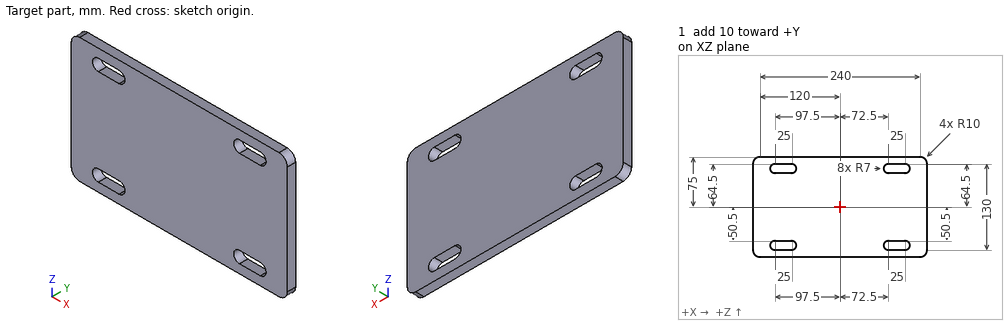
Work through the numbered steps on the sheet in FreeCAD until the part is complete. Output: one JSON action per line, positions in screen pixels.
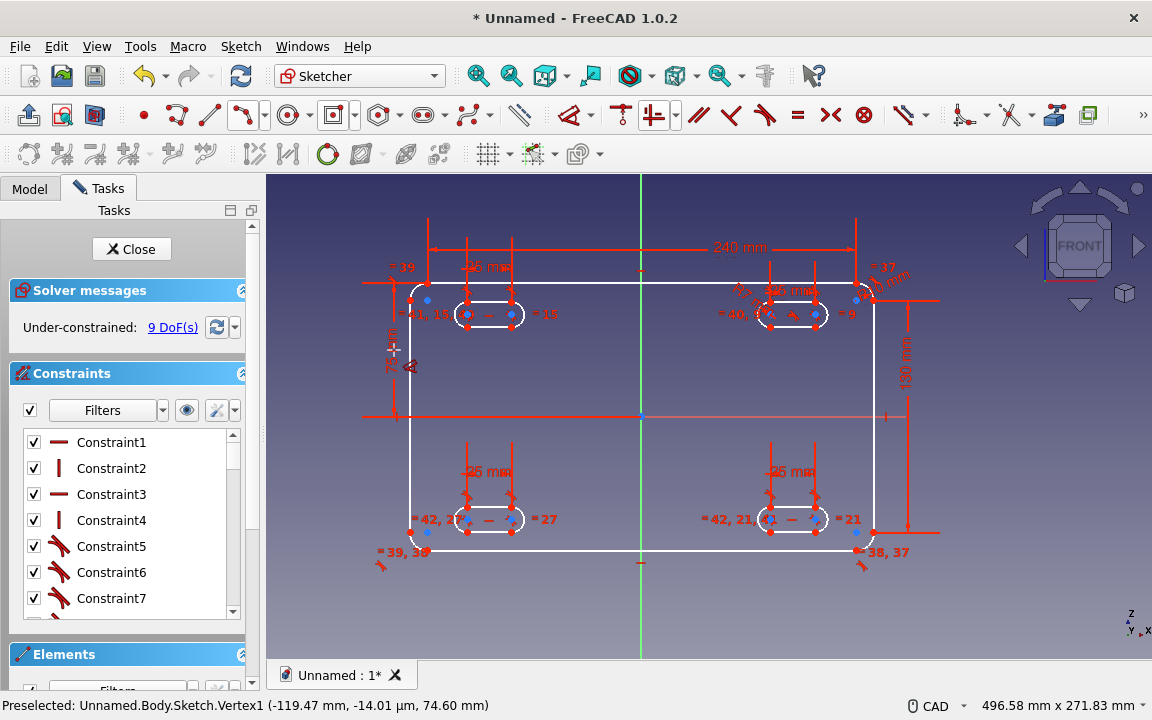
{"action": "left_click", "coordinate": [428, 283]}
{"action": "left_click", "coordinate": [583, 249]}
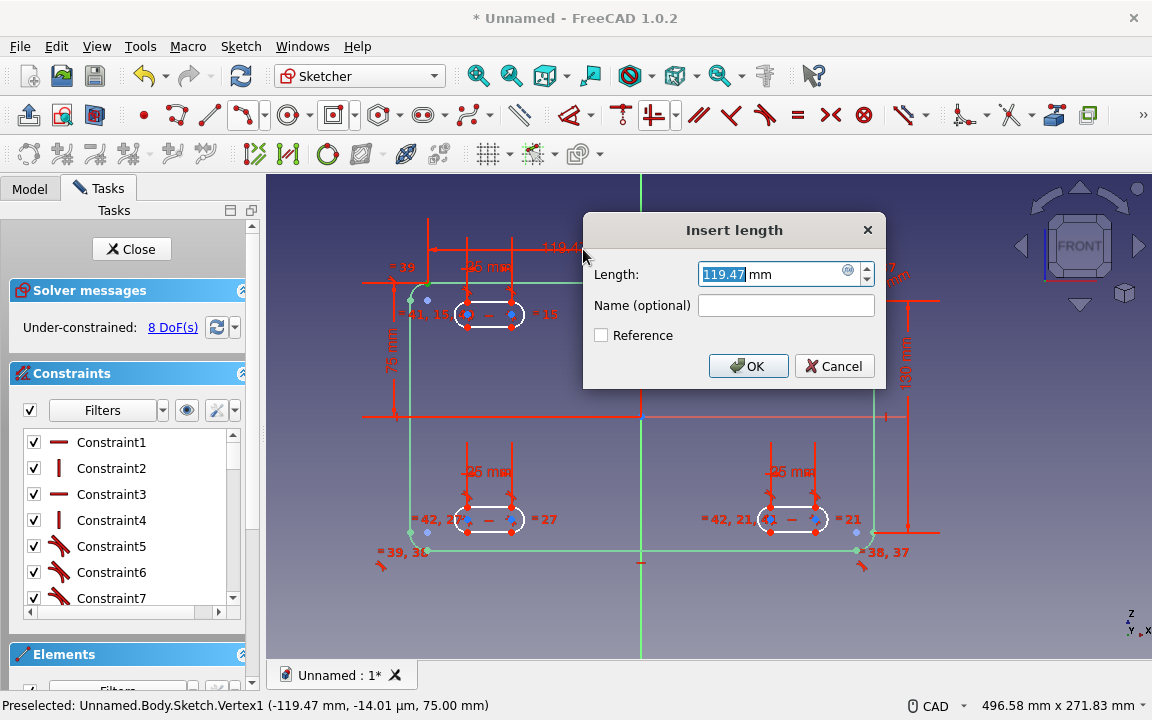
{"action": "type", "text": "120"}
{"action": "key", "text": "Return"}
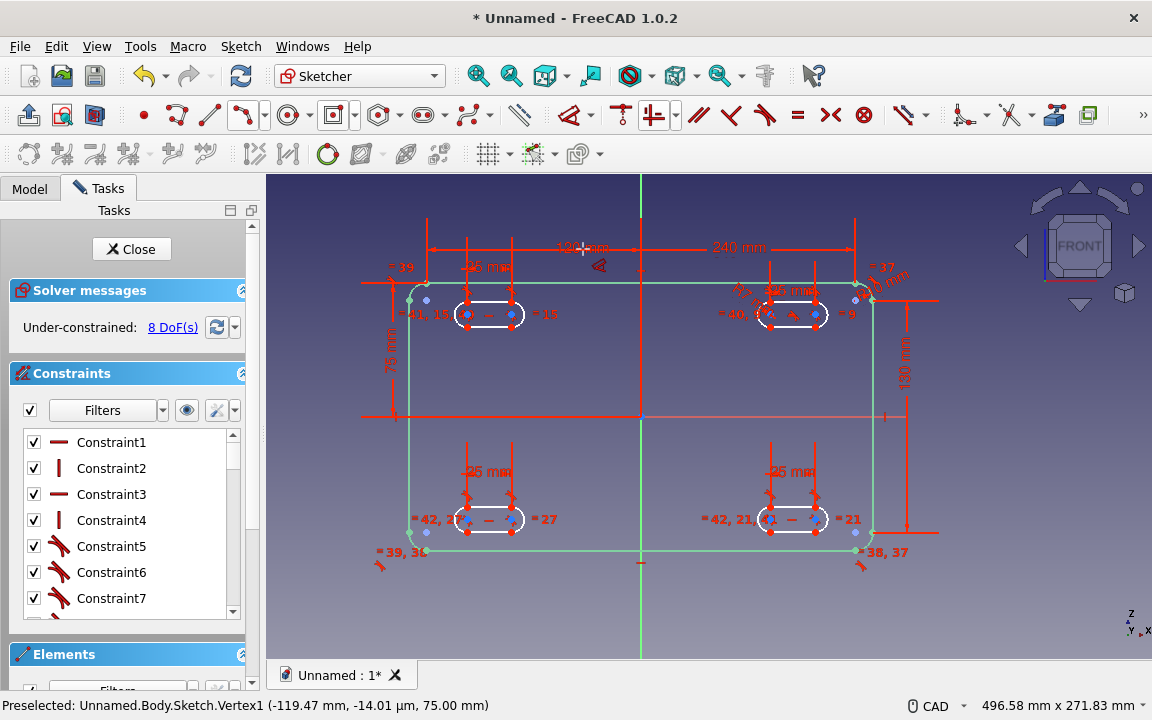
{"action": "left_click", "coordinate": [770, 302]}
{"action": "left_click", "coordinate": [660, 268]}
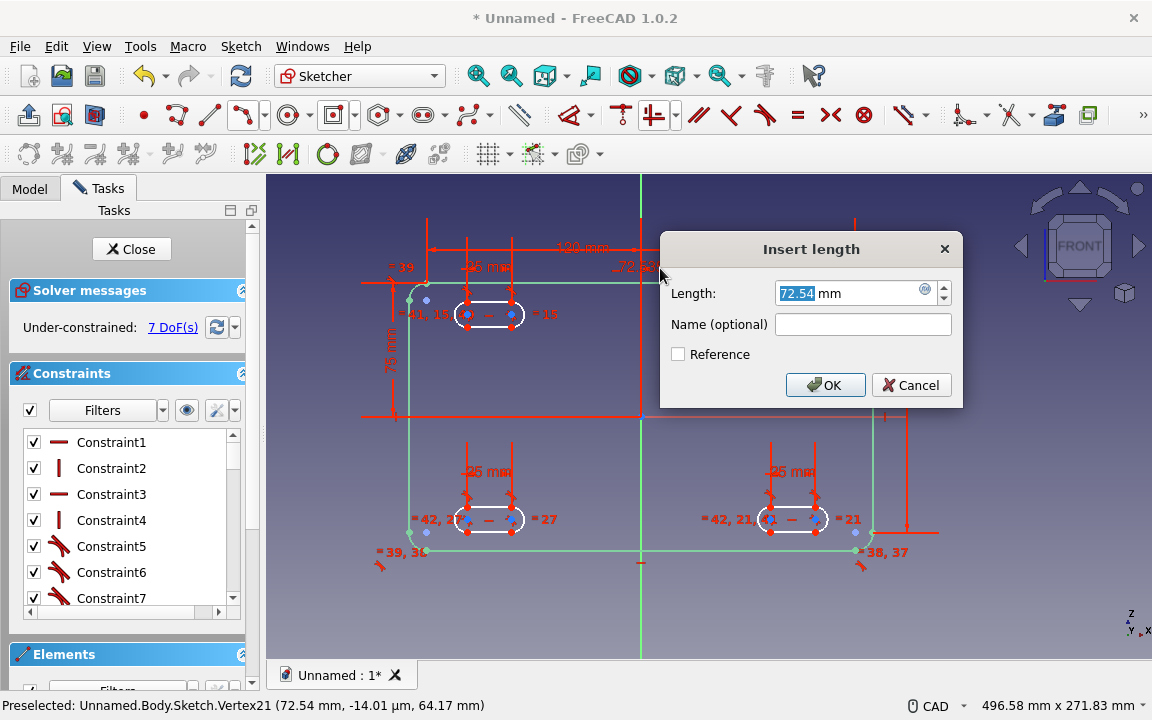
{"action": "type", "text": "72.5"}
{"action": "key", "text": "Return"}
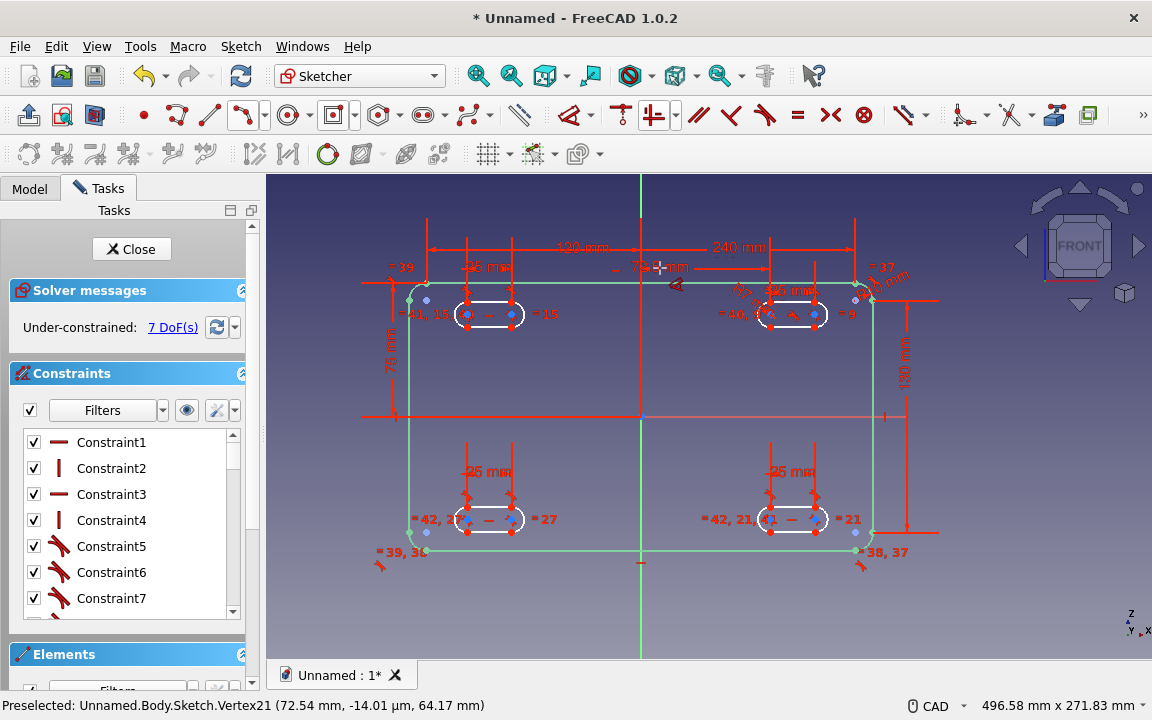
{"action": "left_click", "coordinate": [770, 302]}
{"action": "left_click", "coordinate": [804, 360]}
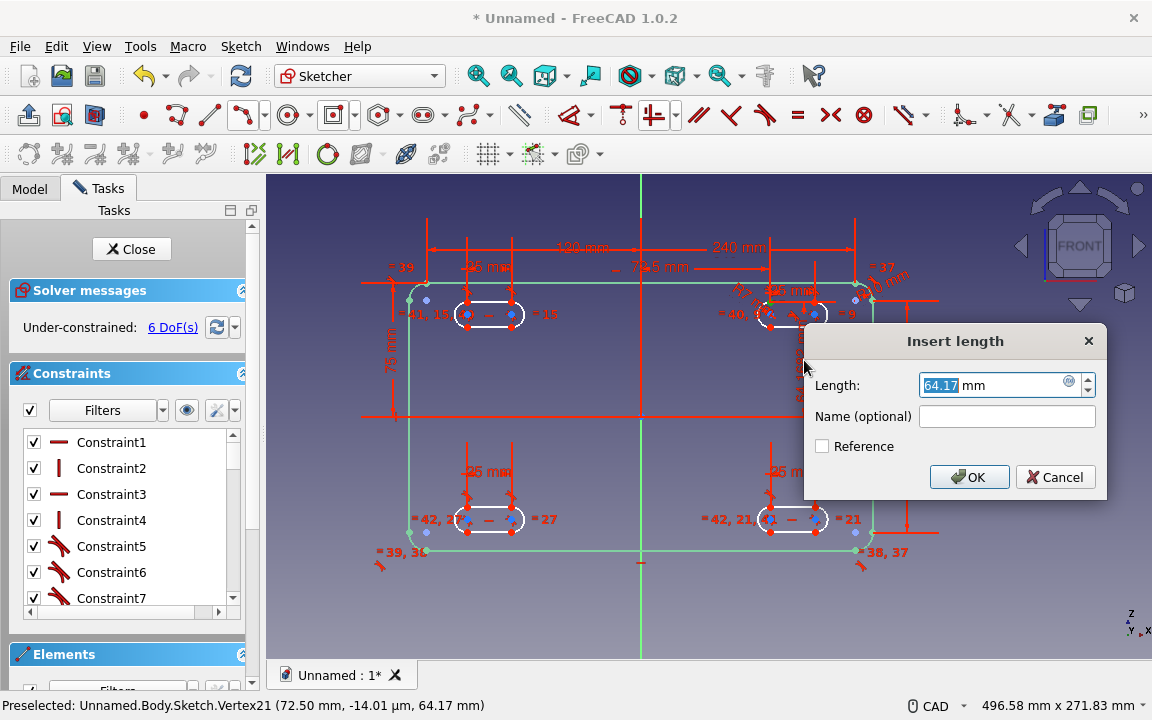
{"action": "type", "text": "64.5"}
{"action": "key", "text": "Return"}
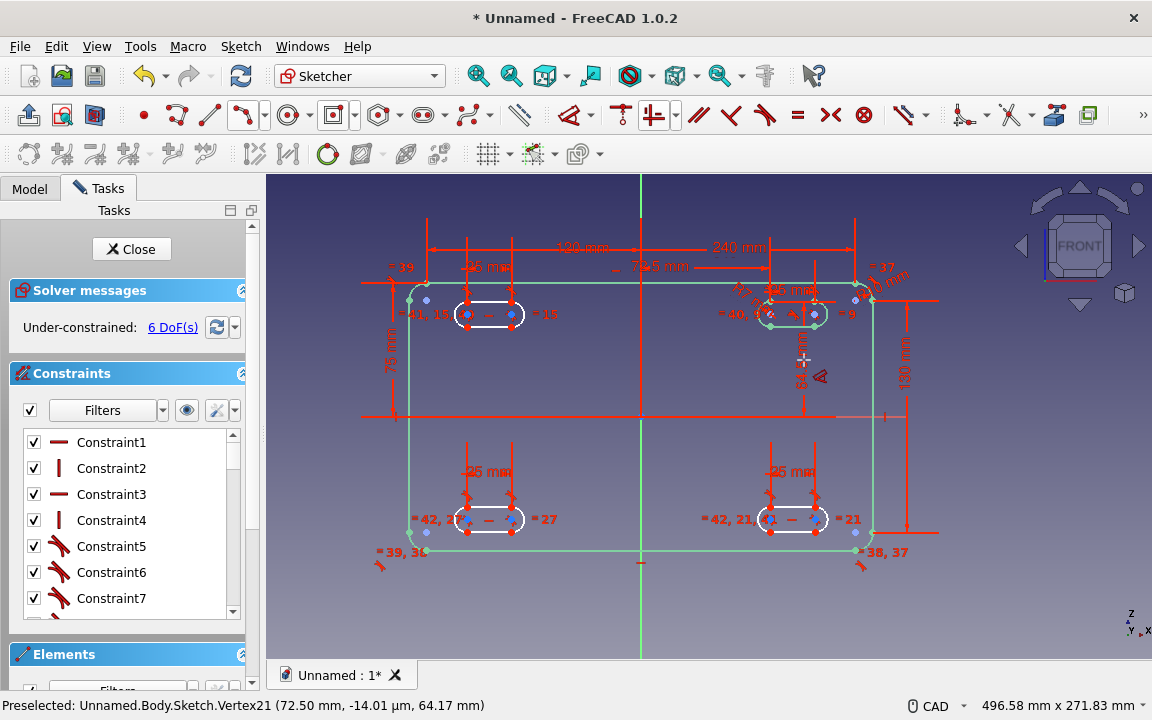
{"action": "left_click", "coordinate": [467, 302]}
{"action": "left_click", "coordinate": [554, 451]}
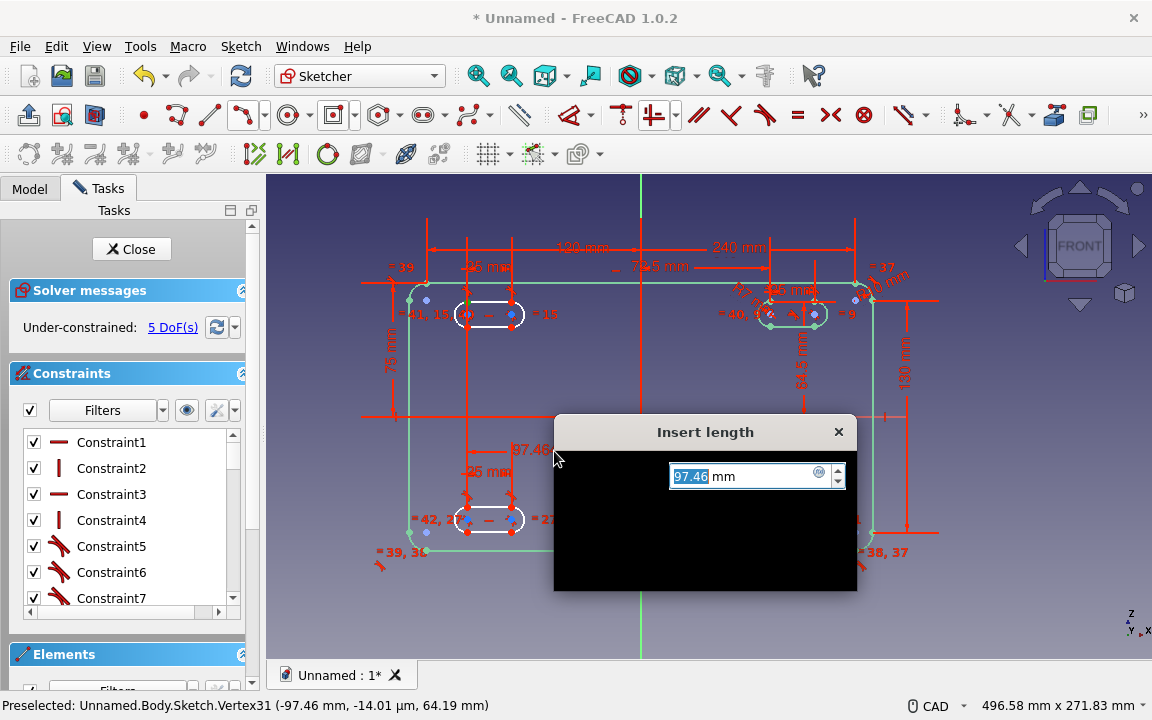
{"action": "type", "text": "97.5"}
{"action": "key", "text": "Return"}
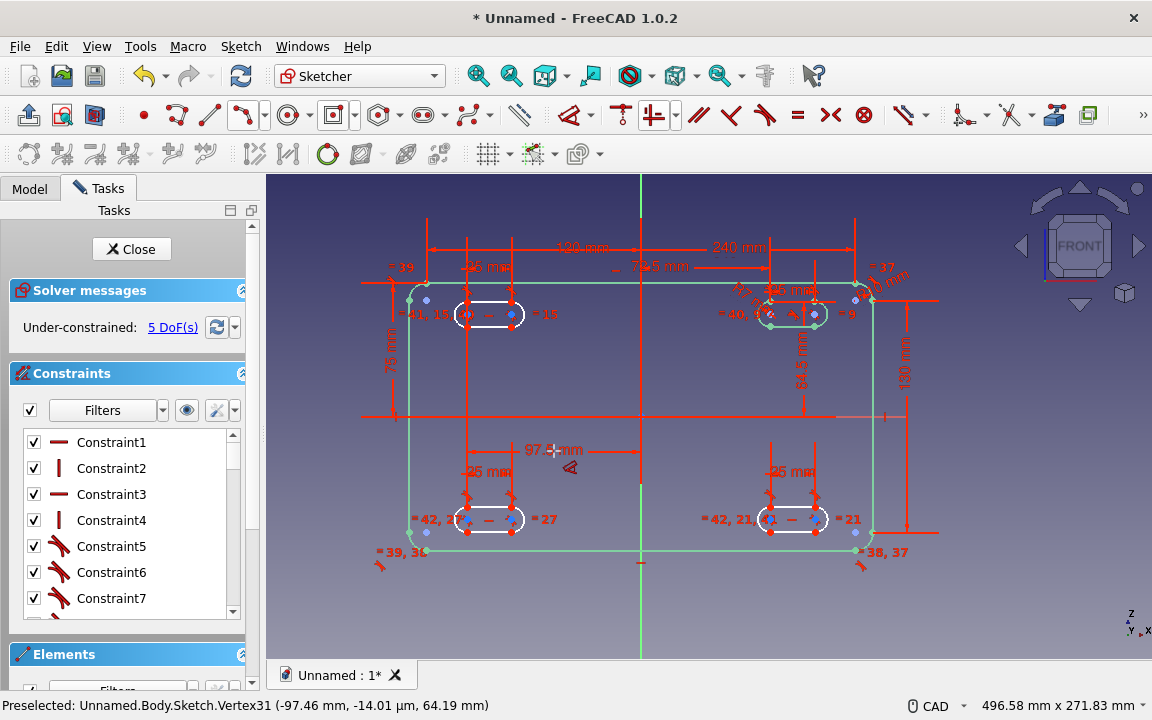
{"action": "left_click", "coordinate": [467, 302]}
{"action": "left_click", "coordinate": [433, 386]}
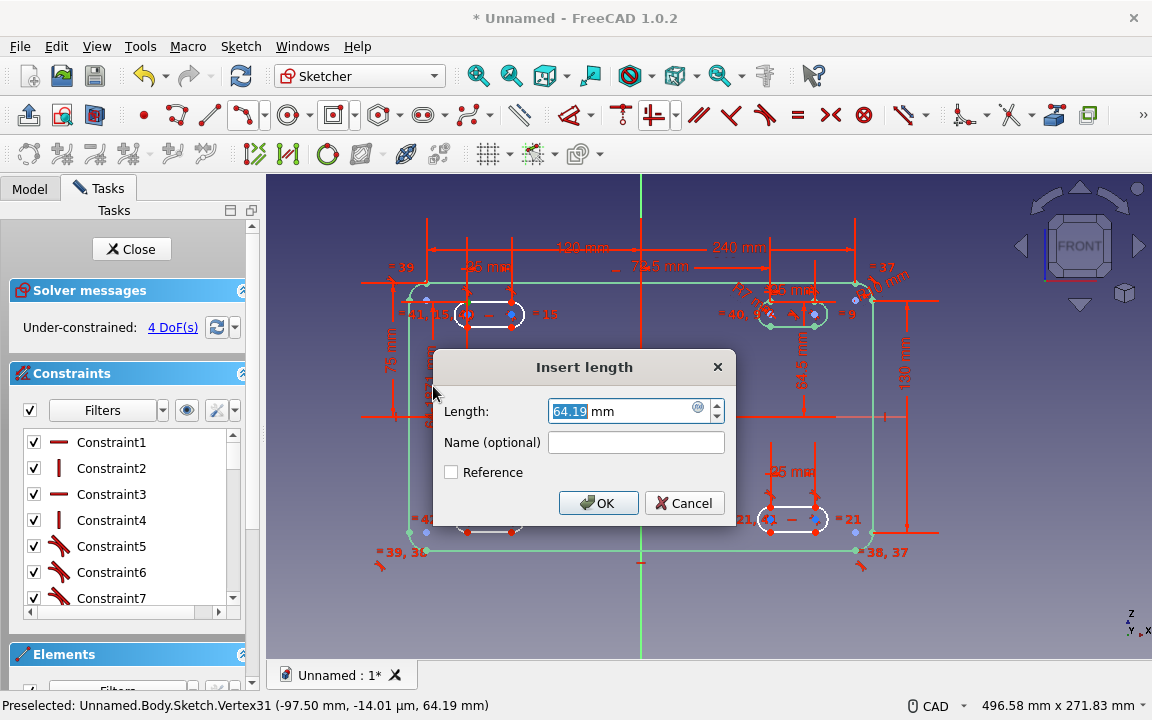
{"action": "type", "text": "64.5"}
{"action": "key", "text": "Return"}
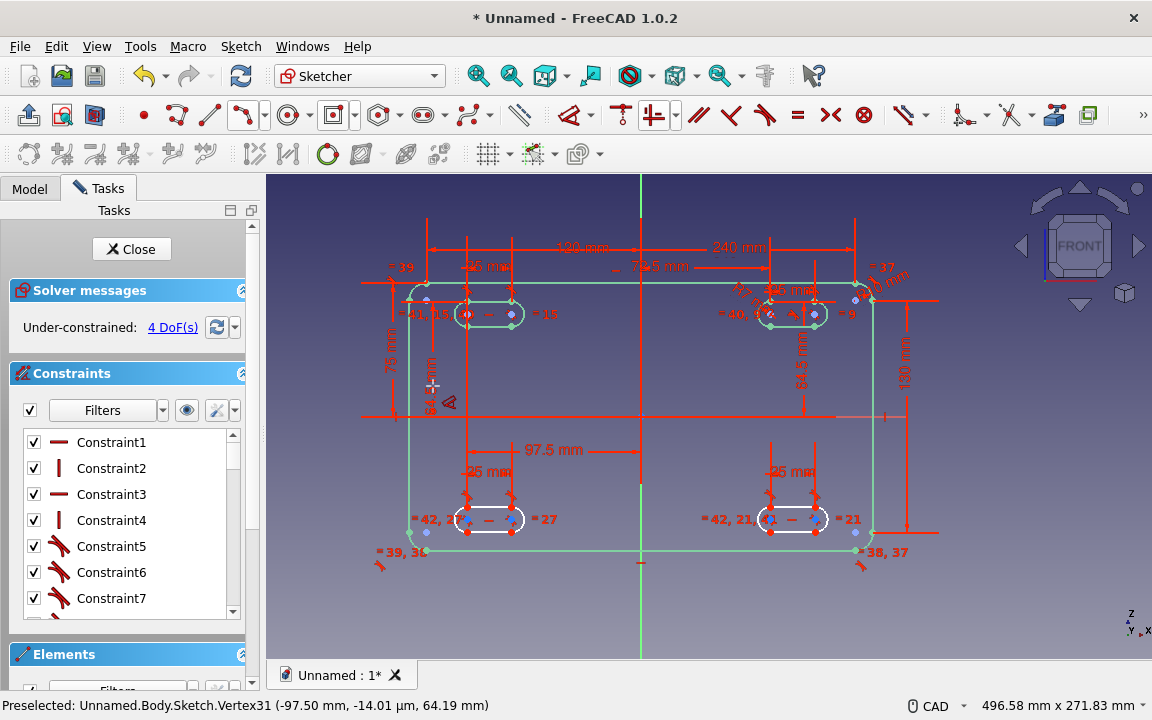
{"action": "left_click", "coordinate": [771, 507]}
{"action": "left_click", "coordinate": [706, 383]}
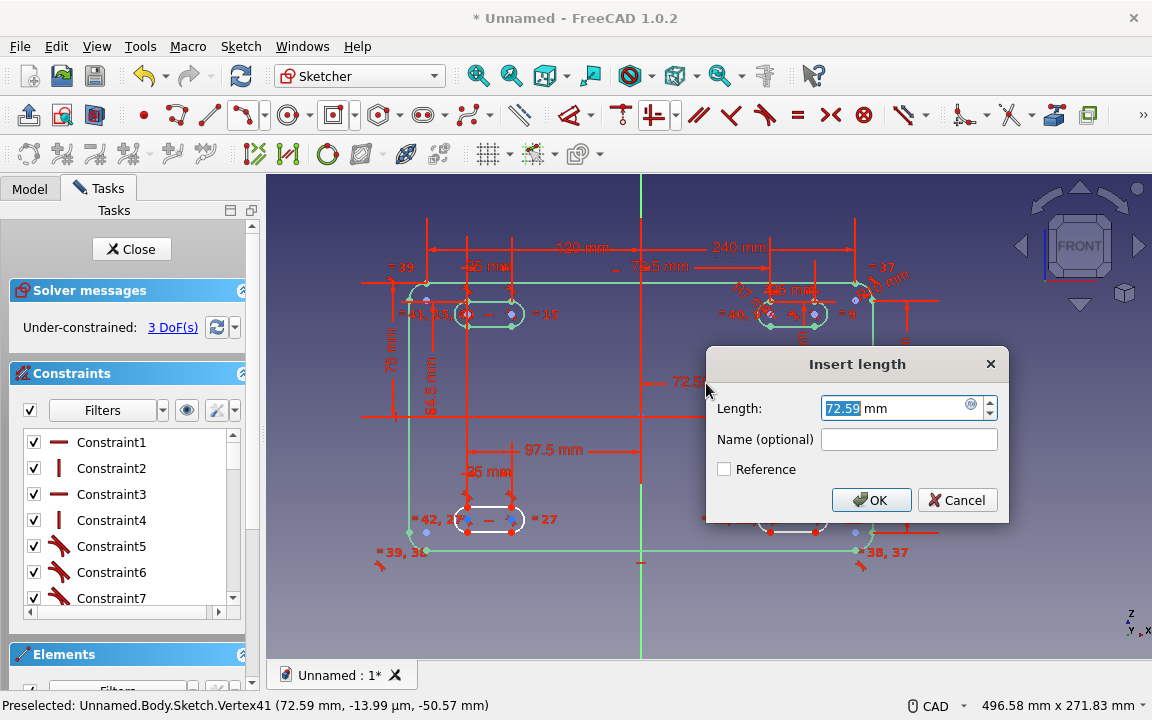
{"action": "type", "text": "72.5"}
{"action": "key", "text": "Return"}